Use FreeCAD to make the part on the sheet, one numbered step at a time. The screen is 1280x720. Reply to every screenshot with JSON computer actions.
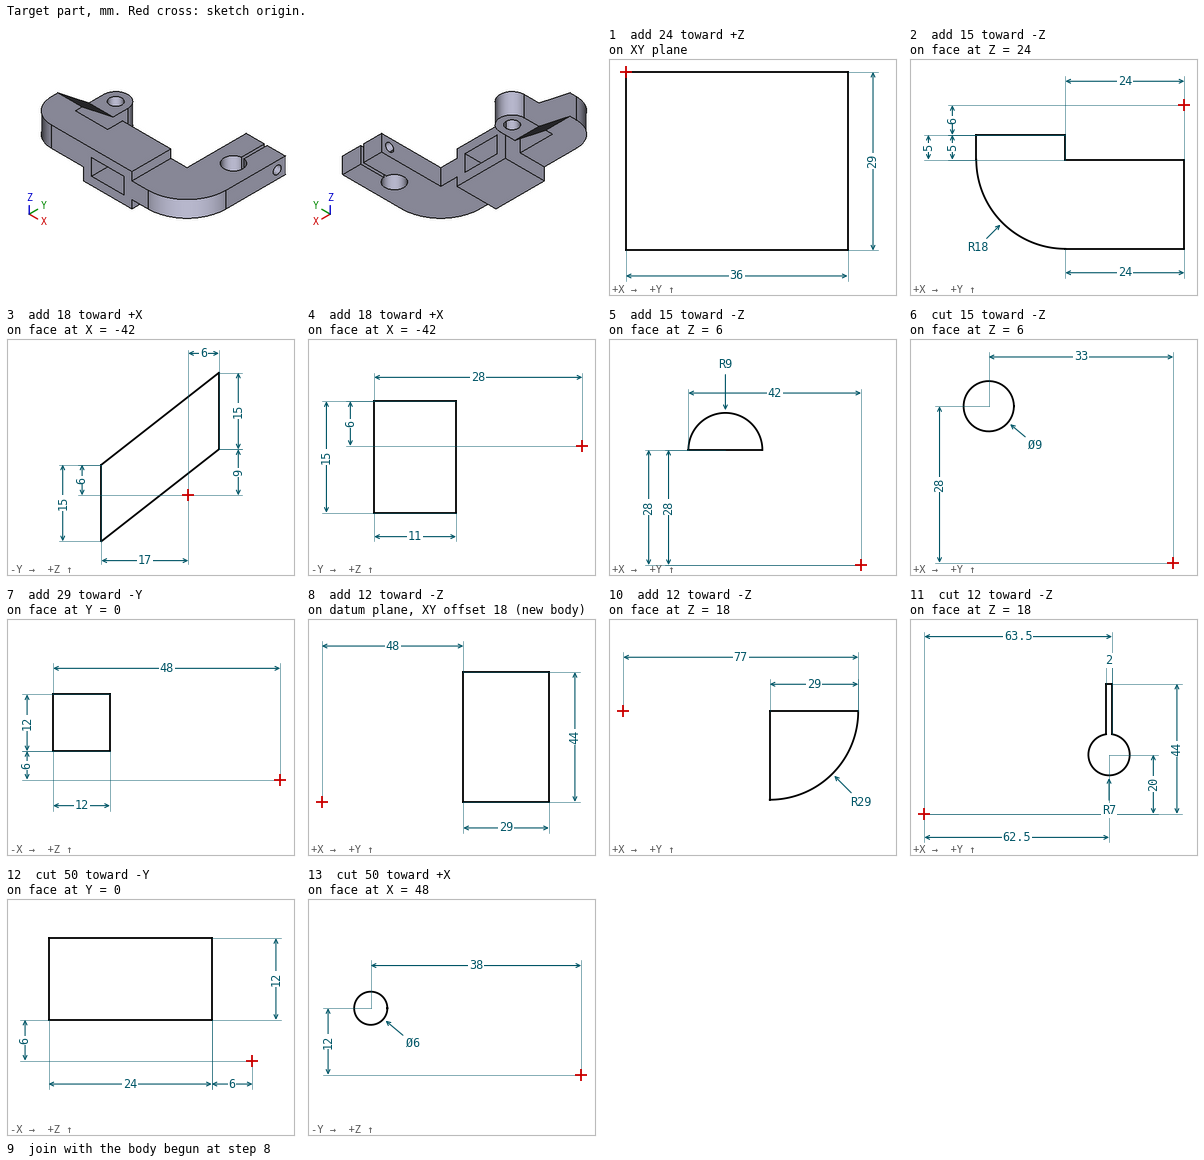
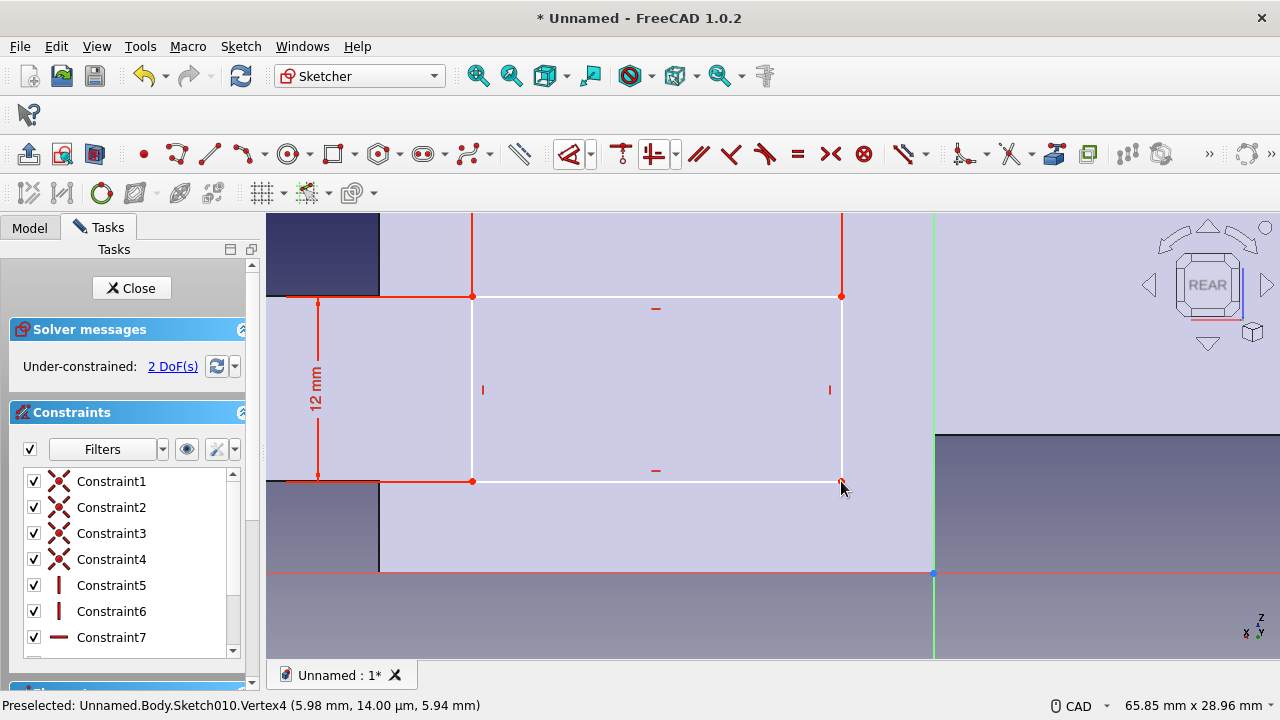
{"action": "left_click", "coordinate": [472, 482]}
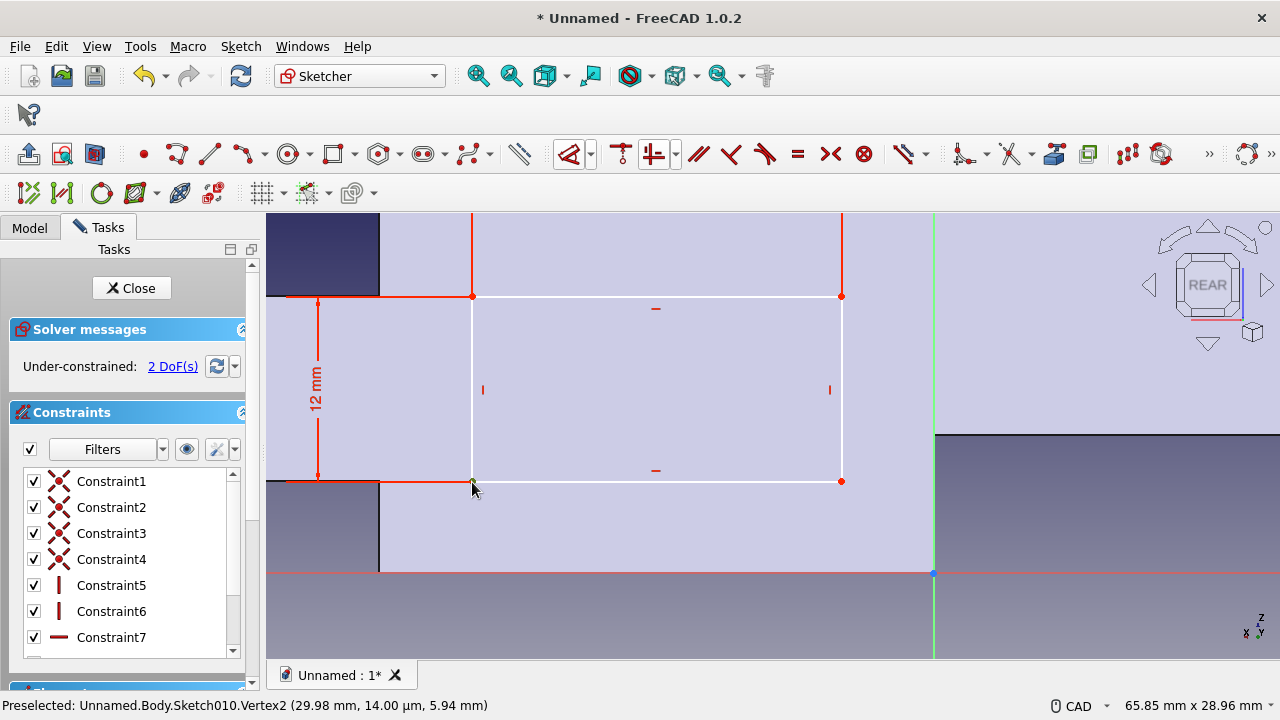
{"action": "key", "text": "i"}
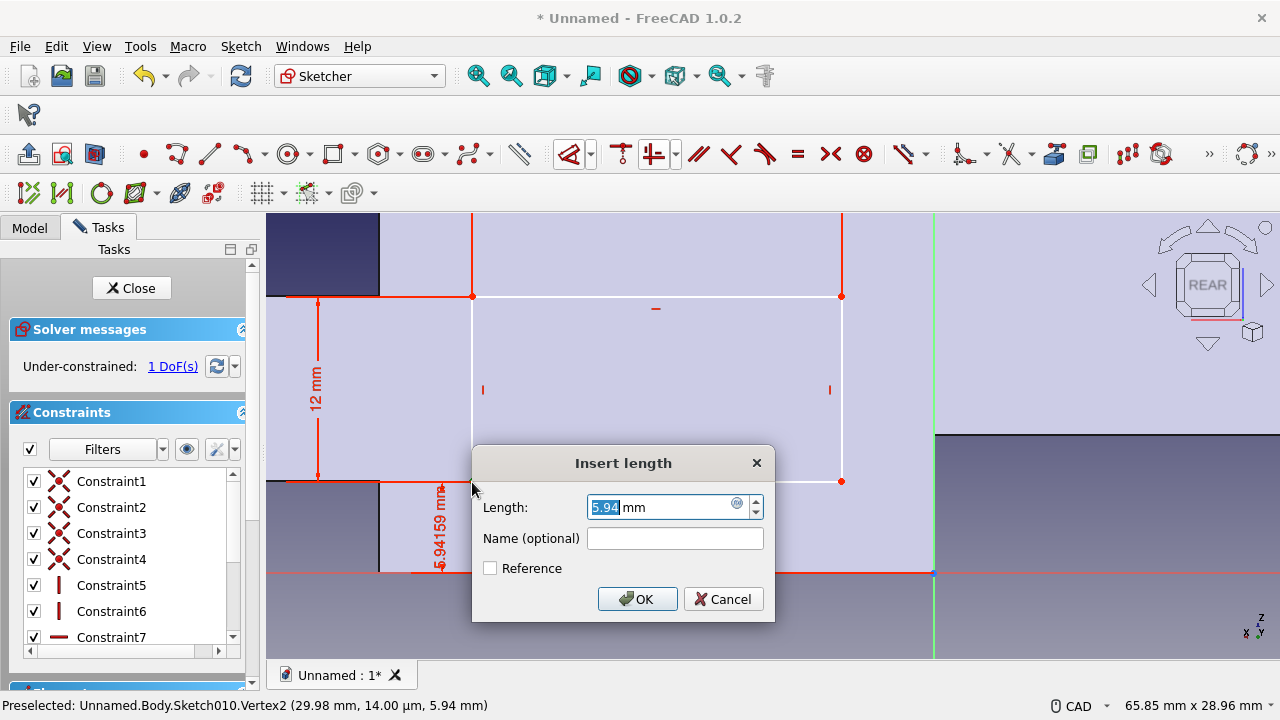
{"action": "type", "text": "6"}
{"action": "key", "text": "Return"}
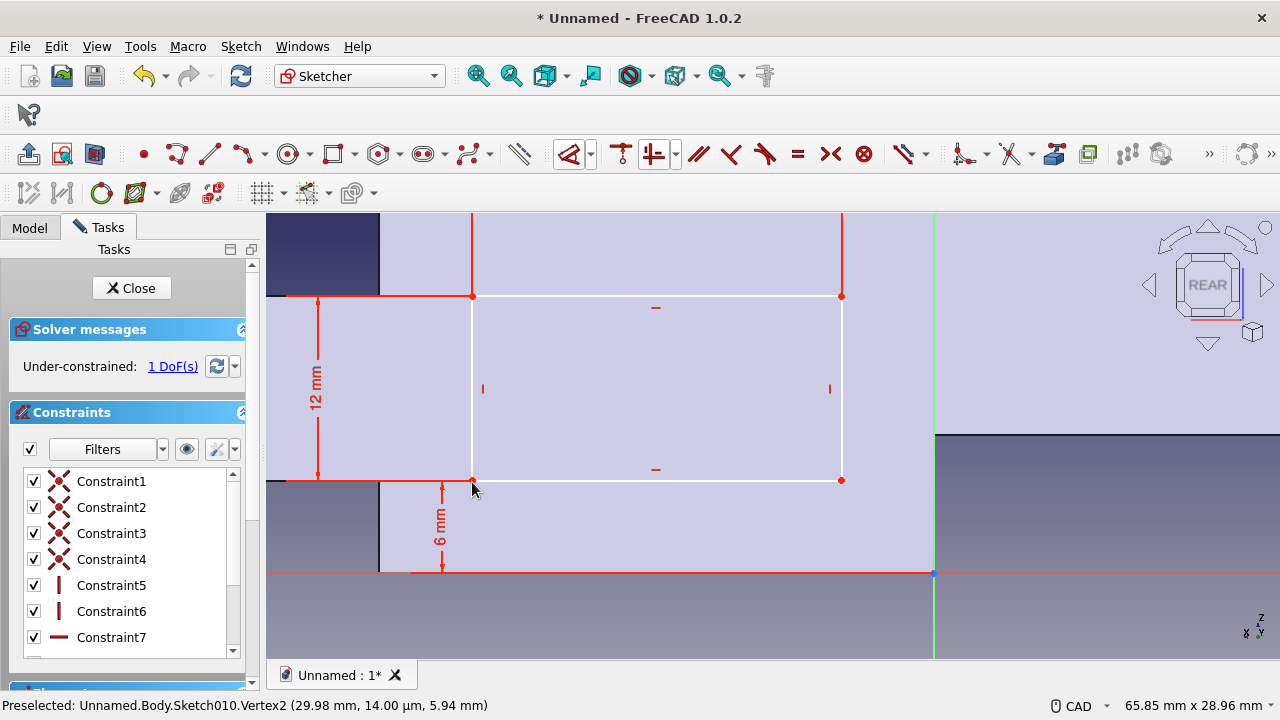
{"action": "left_click", "coordinate": [842, 481]}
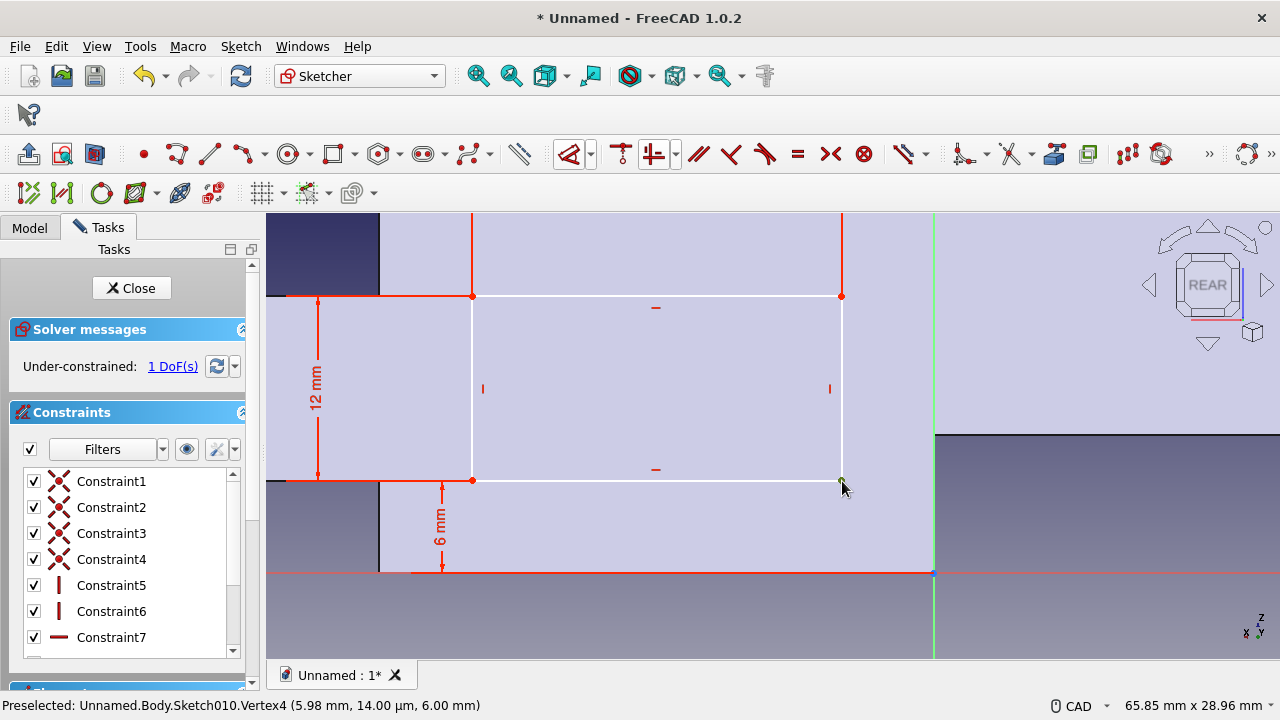
{"action": "key", "text": "l"}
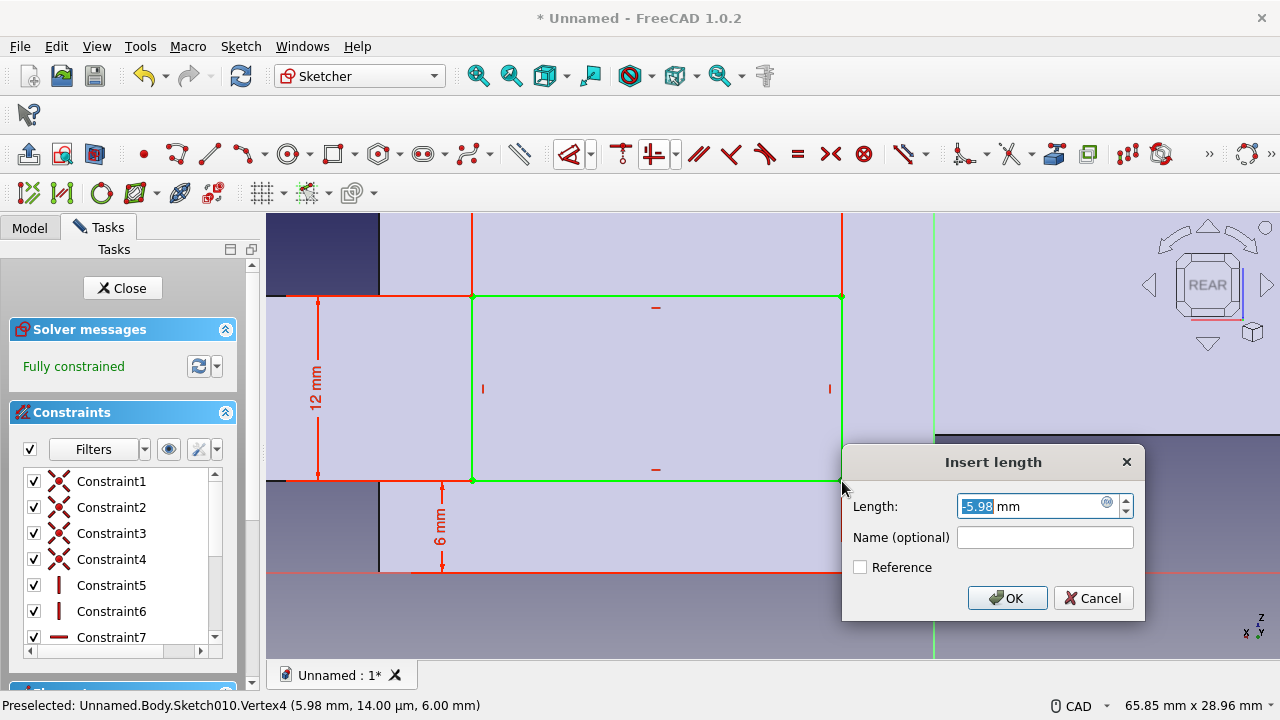
{"action": "type", "text": "-6"}
{"action": "key", "text": "Return"}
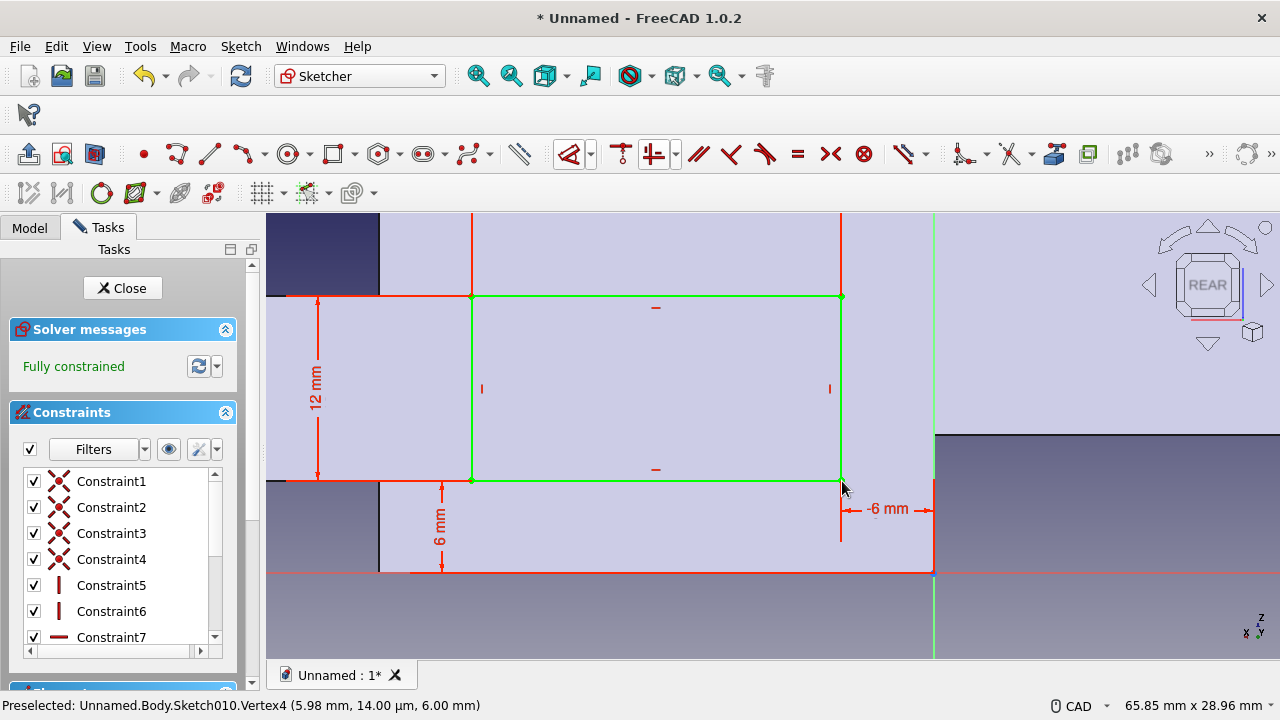
{"action": "left_click", "coordinate": [123, 288]}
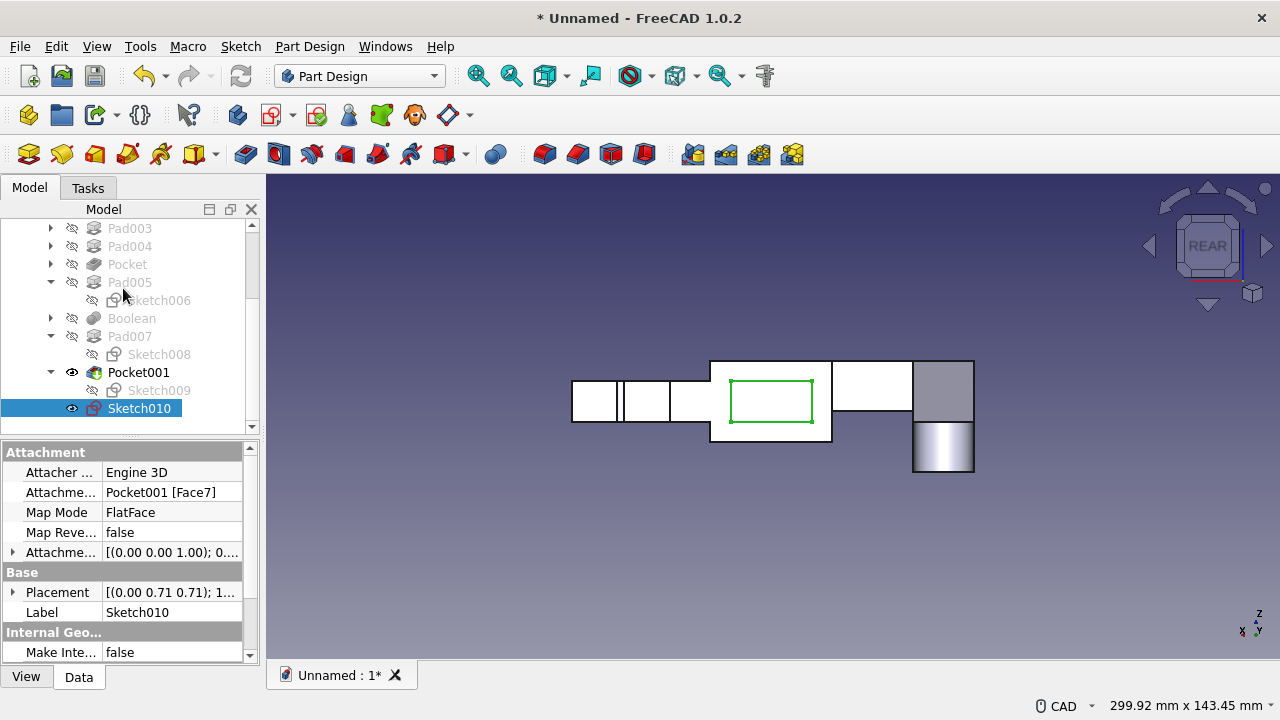
{"action": "left_click", "coordinate": [246, 154]}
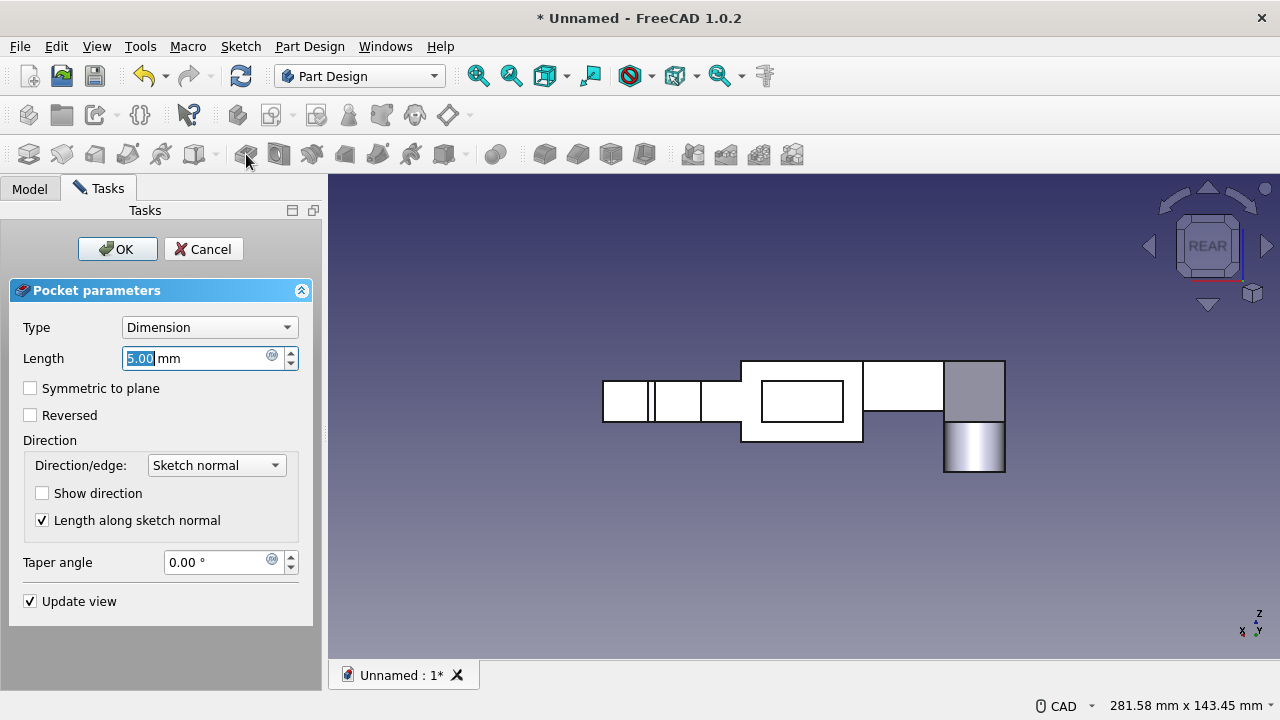
{"action": "type", "text": "50"}
{"action": "key", "text": "Tab"}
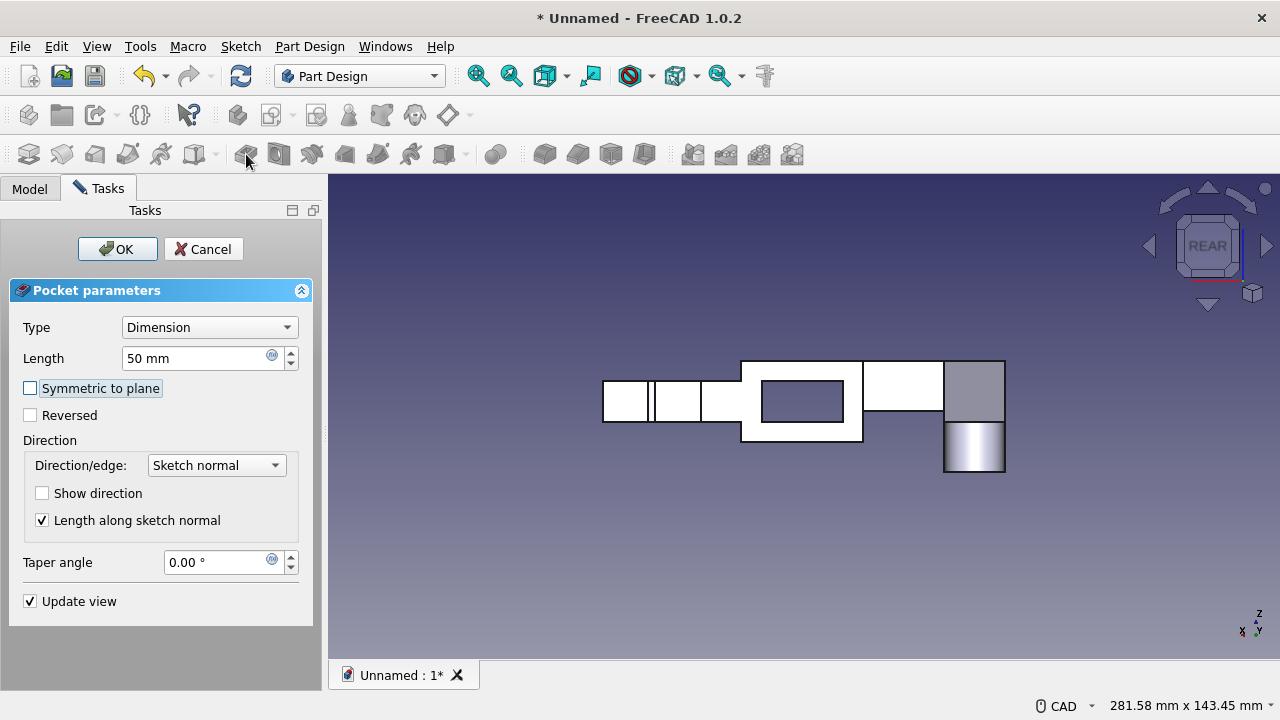
{"action": "left_click", "coordinate": [118, 249]}